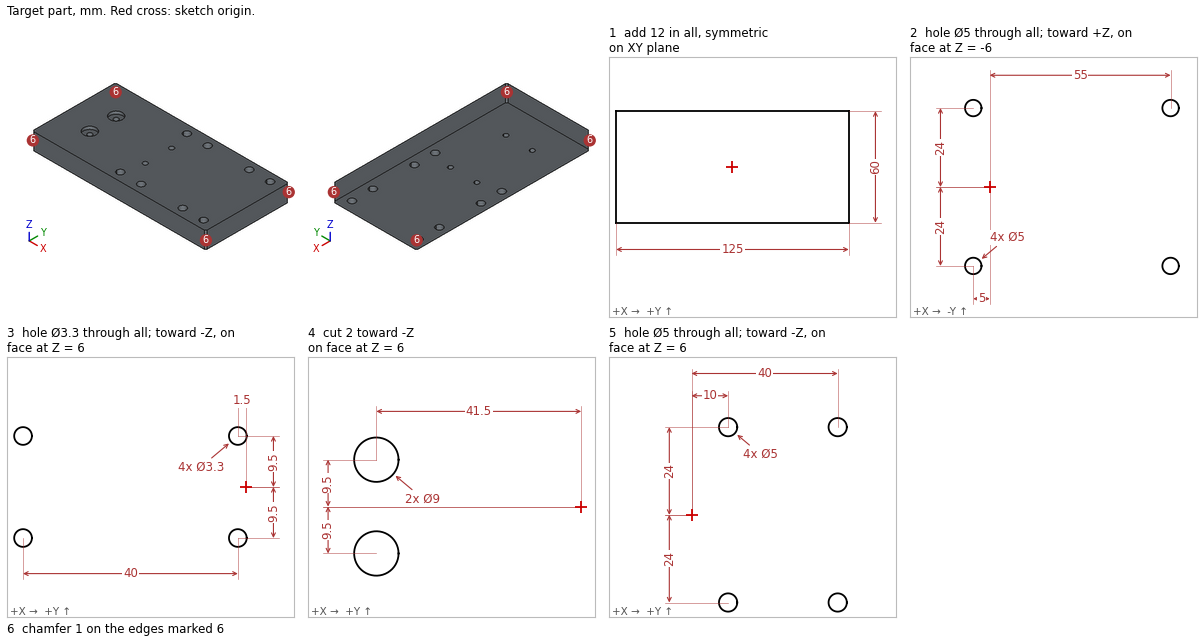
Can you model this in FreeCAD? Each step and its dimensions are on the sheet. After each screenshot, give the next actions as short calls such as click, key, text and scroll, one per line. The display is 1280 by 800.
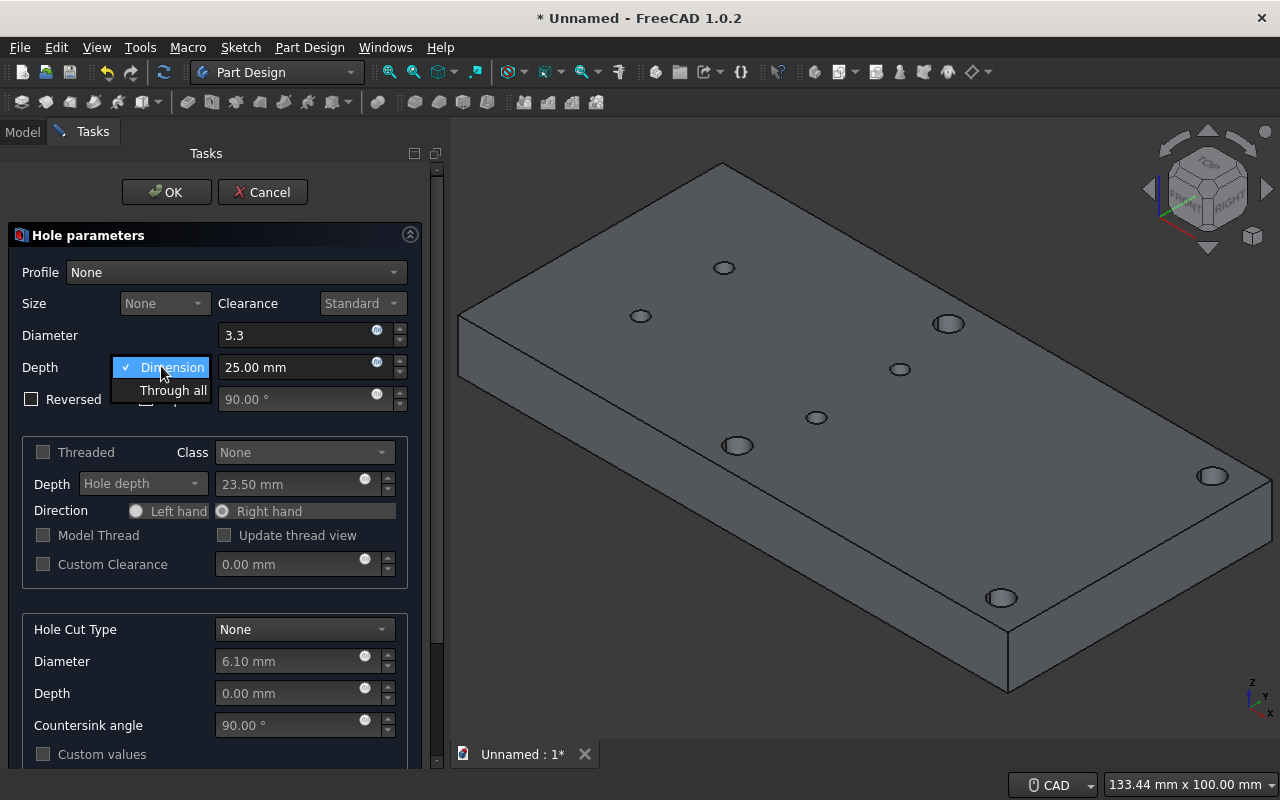
click(160, 390)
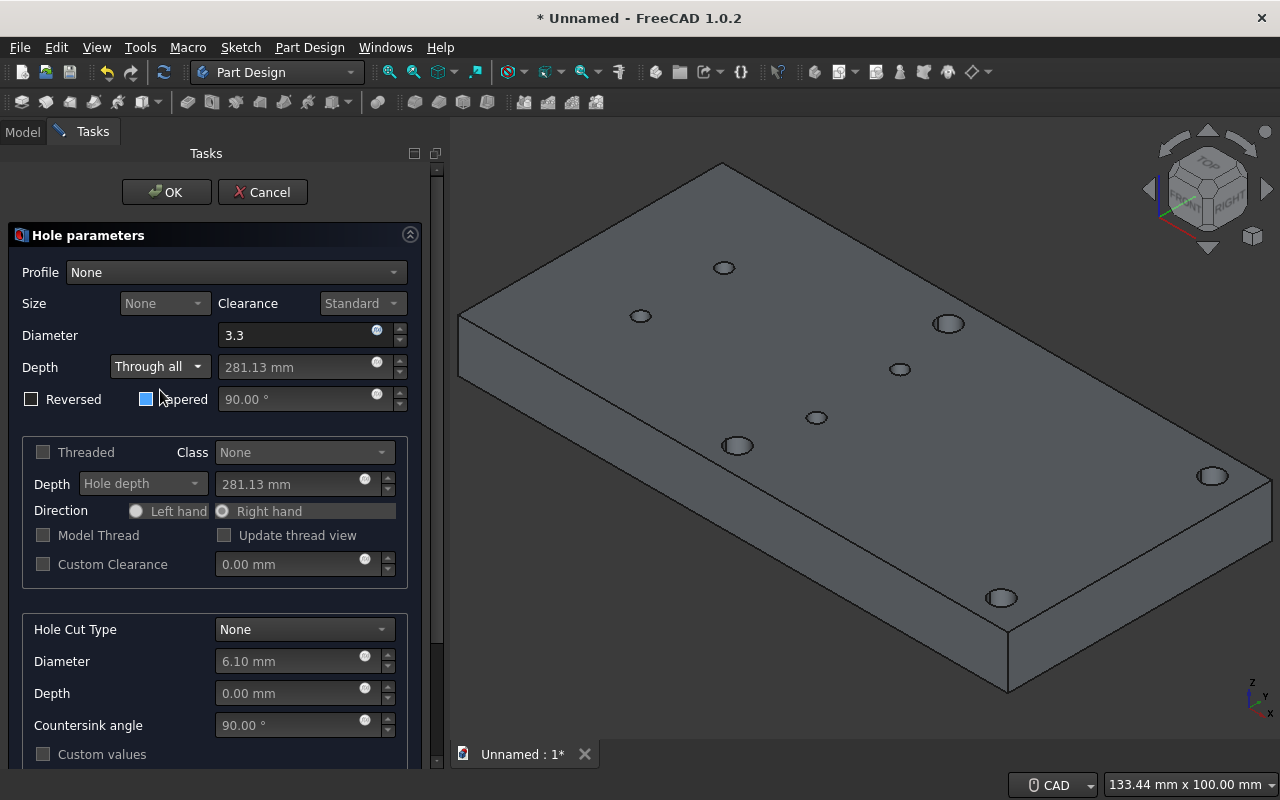
click(167, 192)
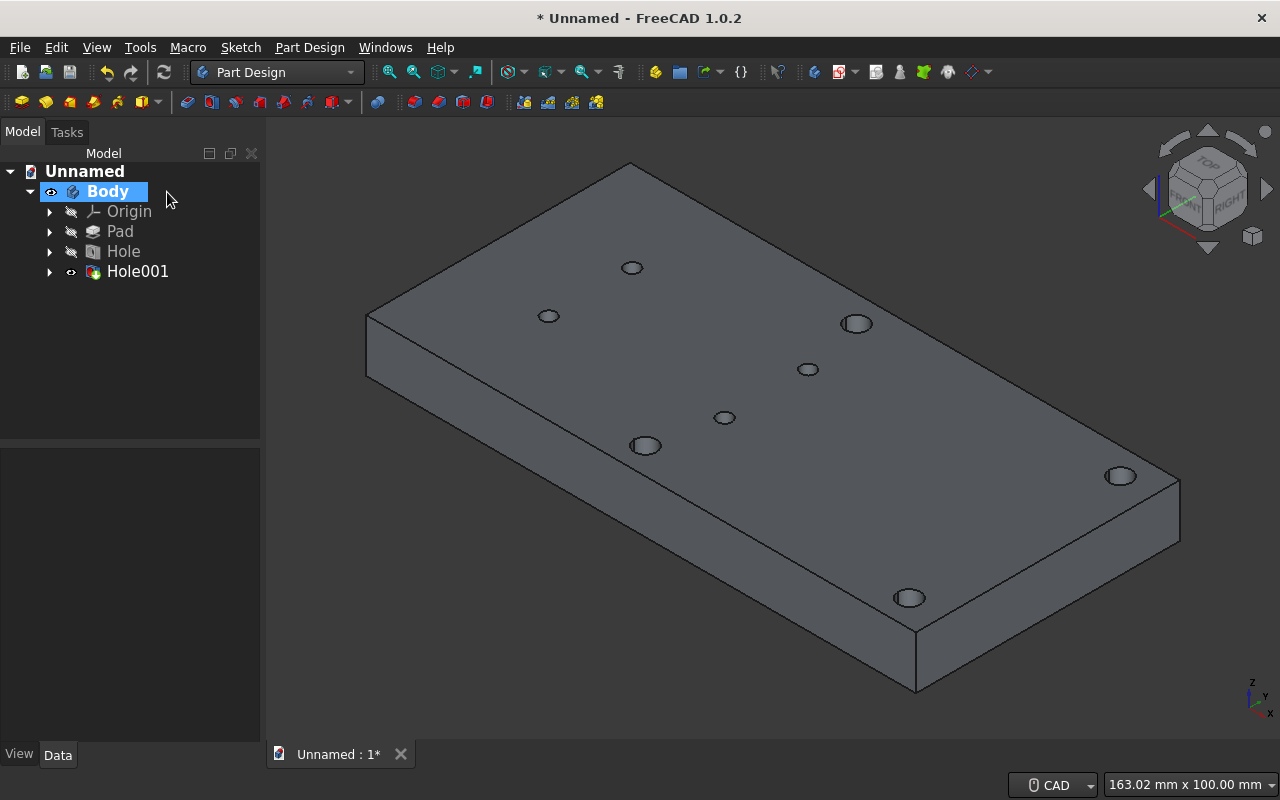
click(930, 487)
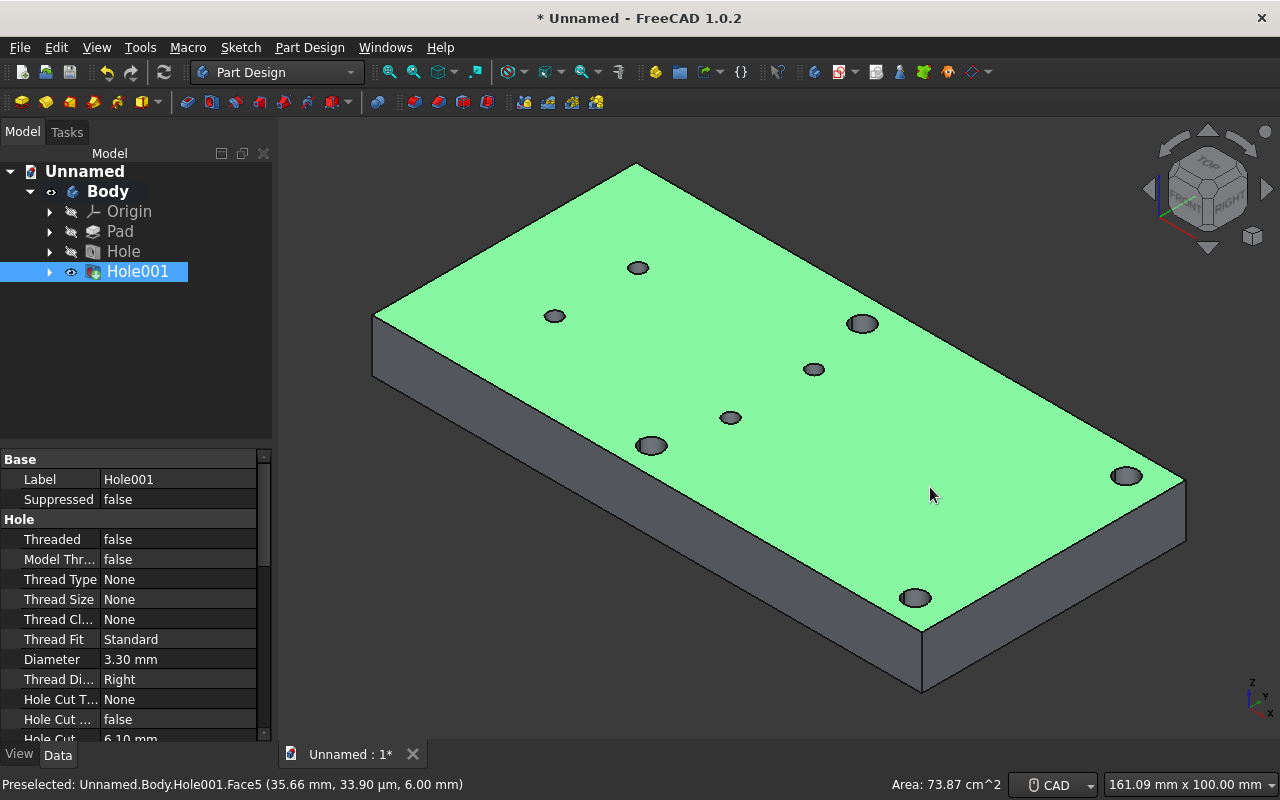
click(840, 72)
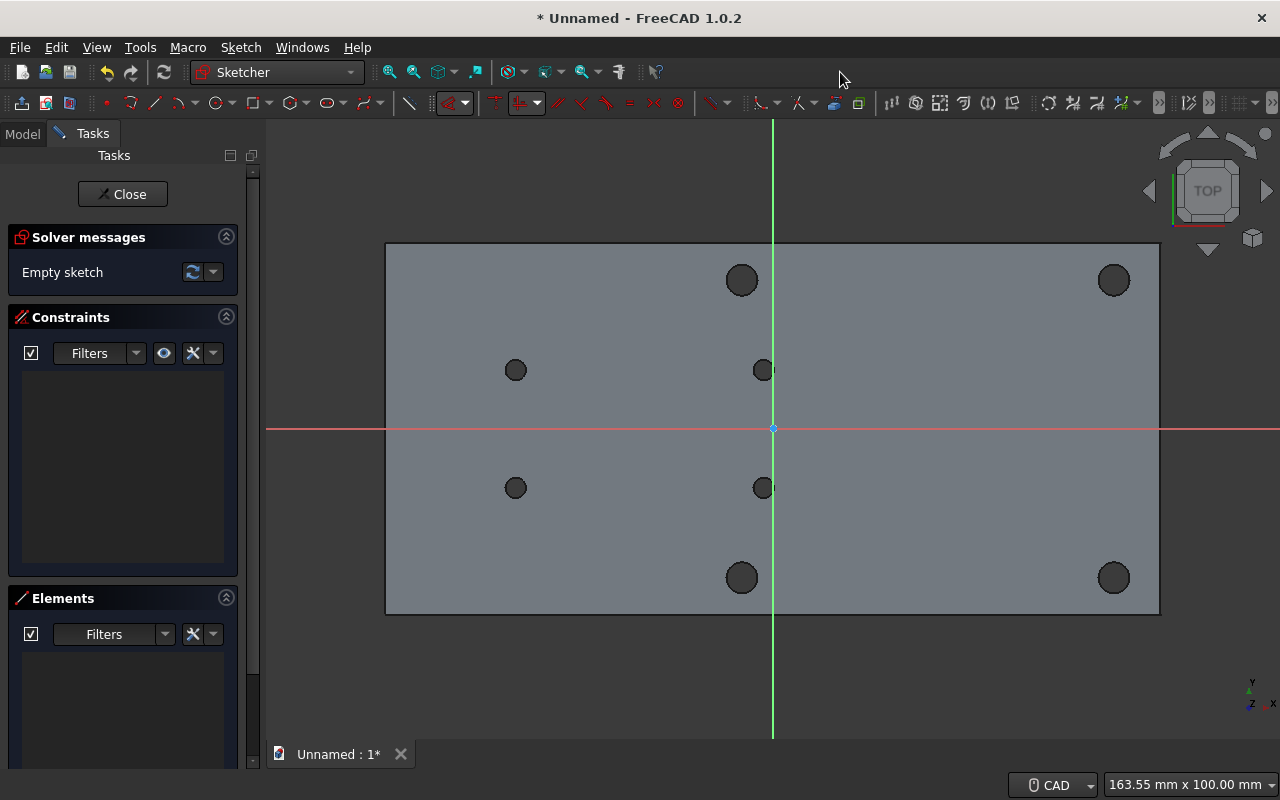
scroll(570, 429, up, 4)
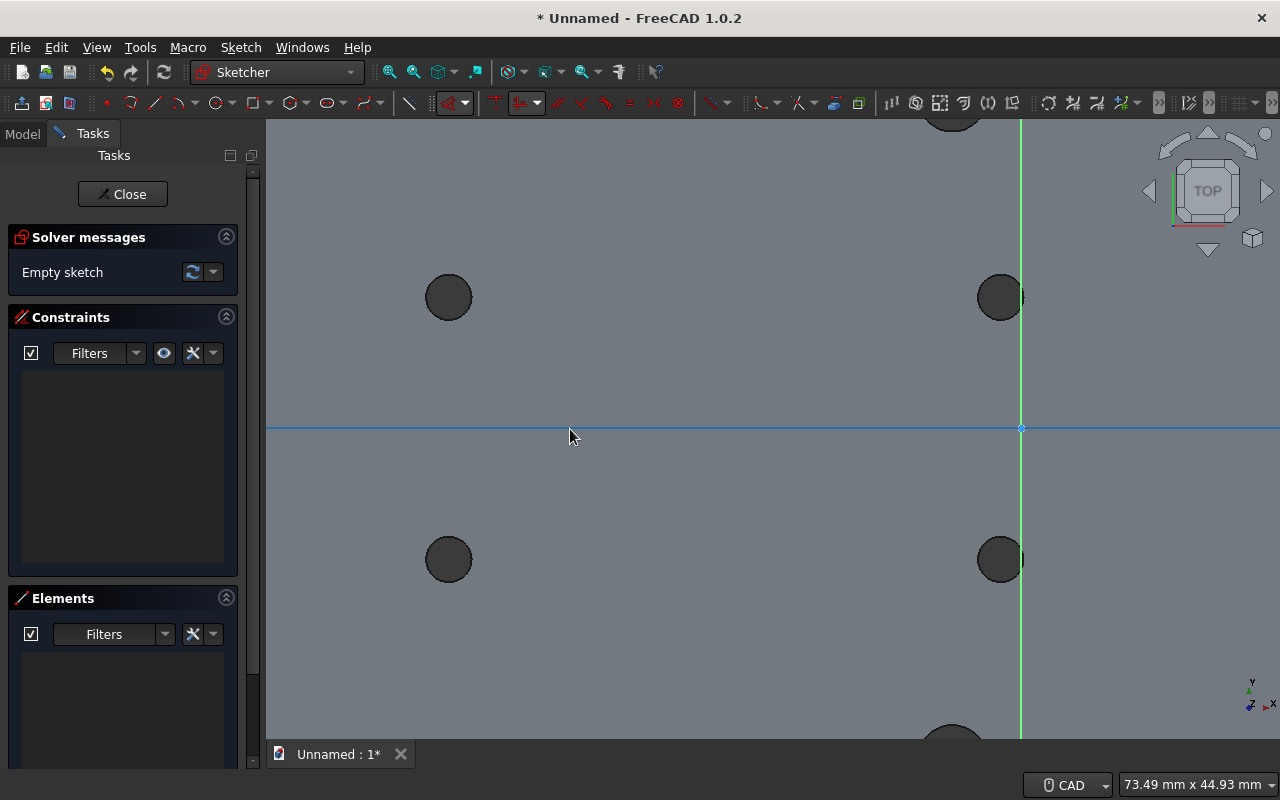
key(g)
key(c)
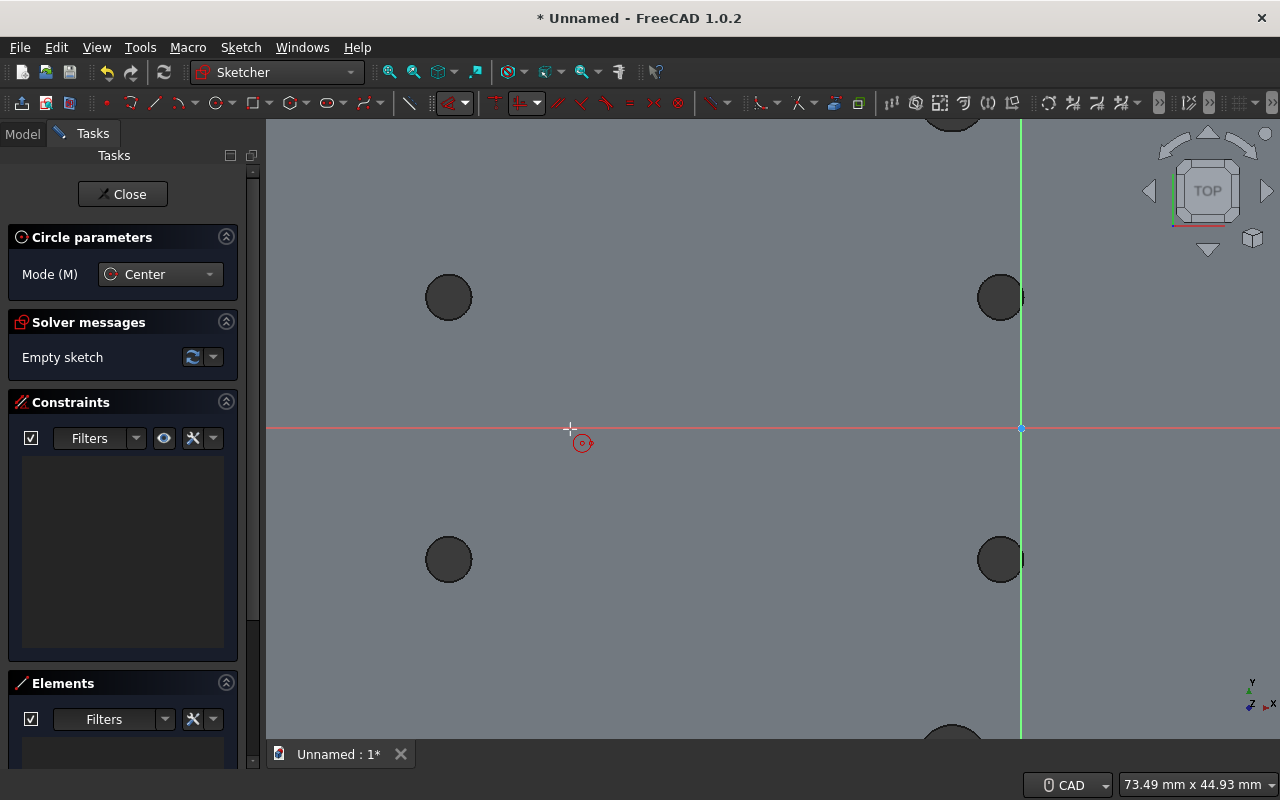
click(449, 297)
click(493, 253)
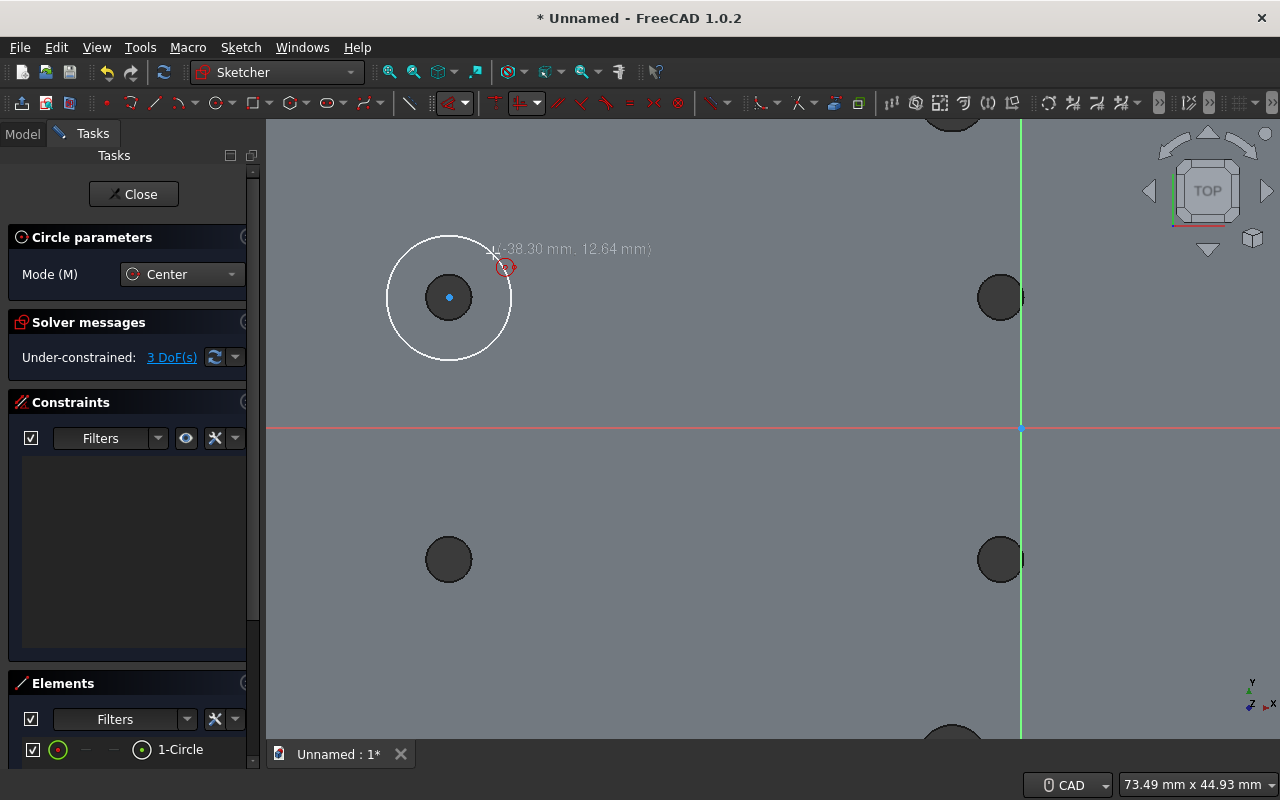
click(449, 559)
click(493, 516)
key(Escape)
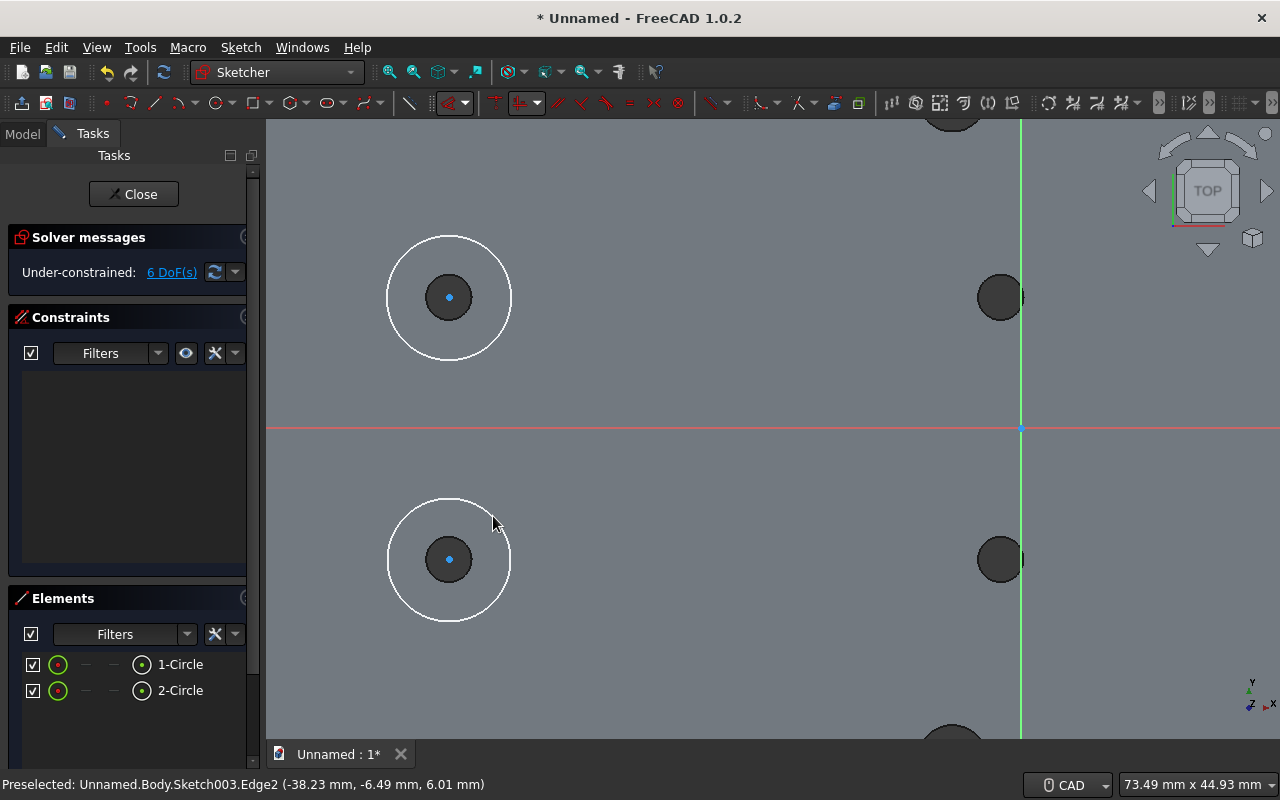
click(493, 254)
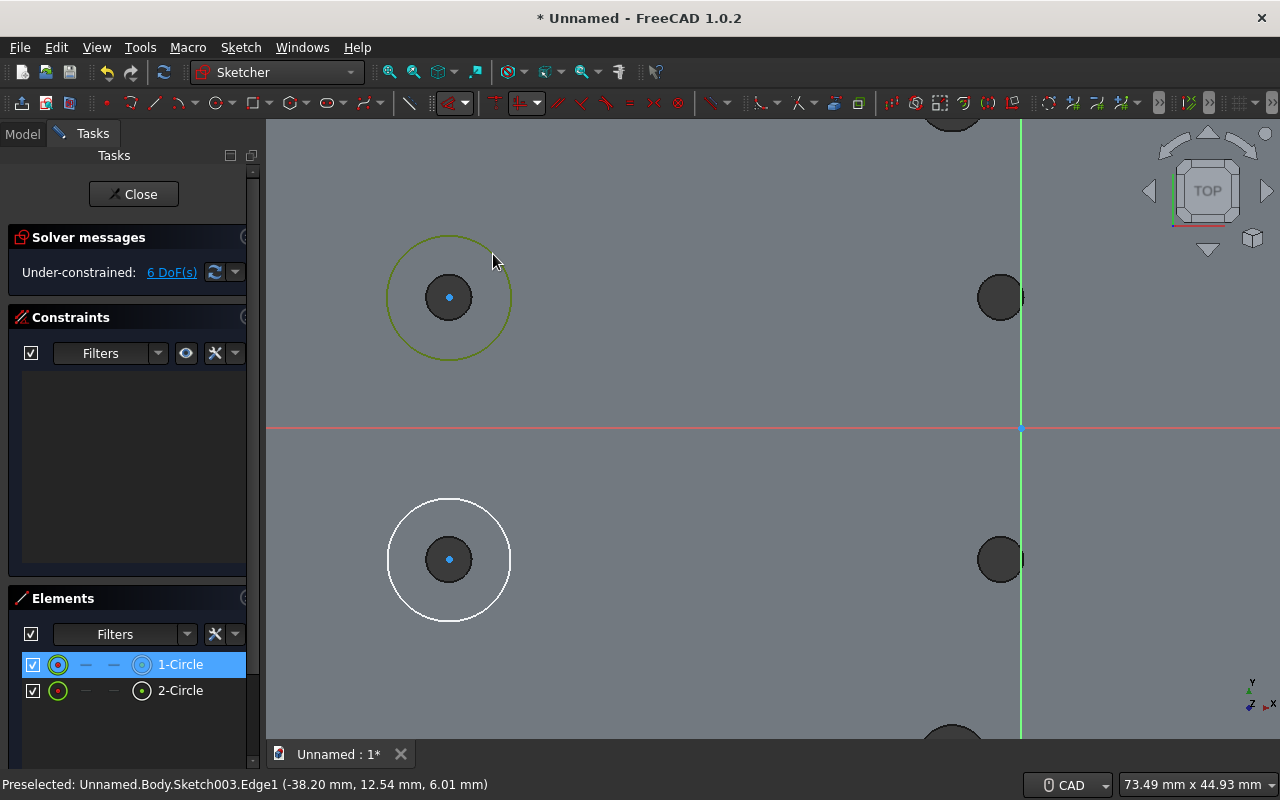
click(492, 516)